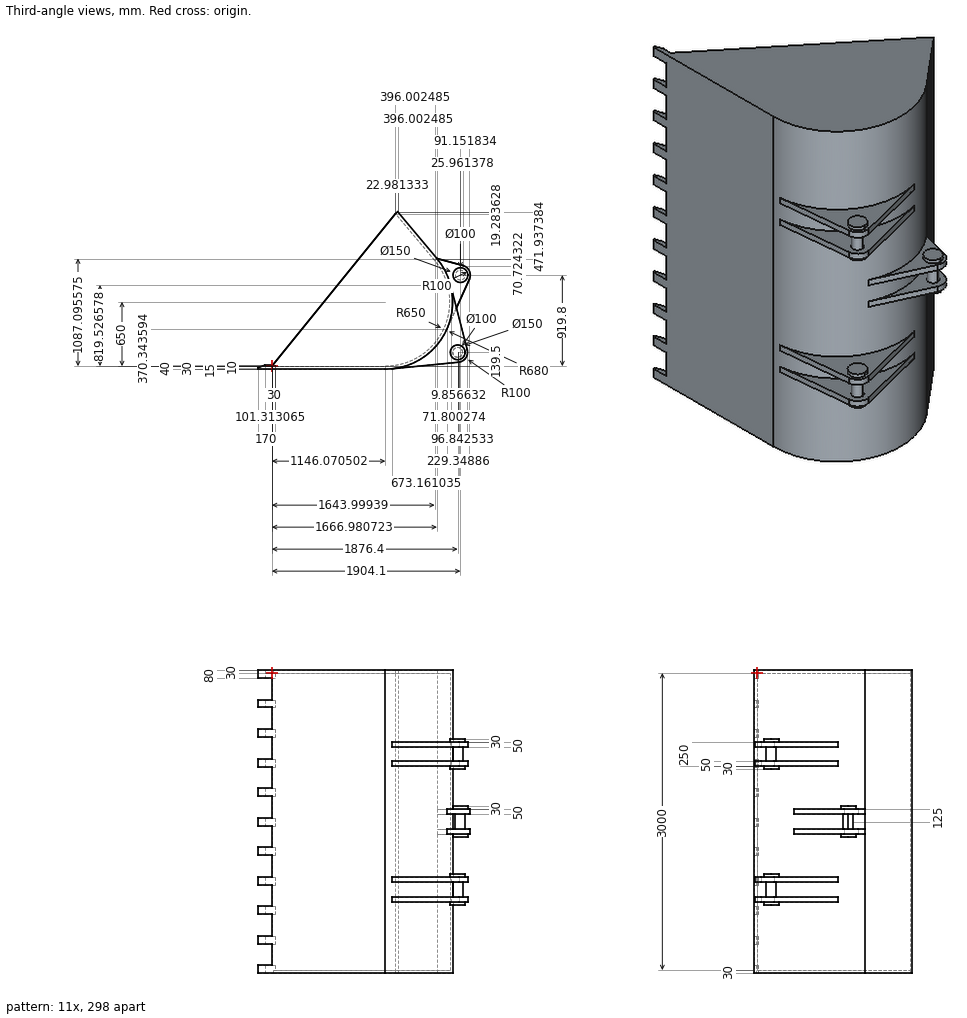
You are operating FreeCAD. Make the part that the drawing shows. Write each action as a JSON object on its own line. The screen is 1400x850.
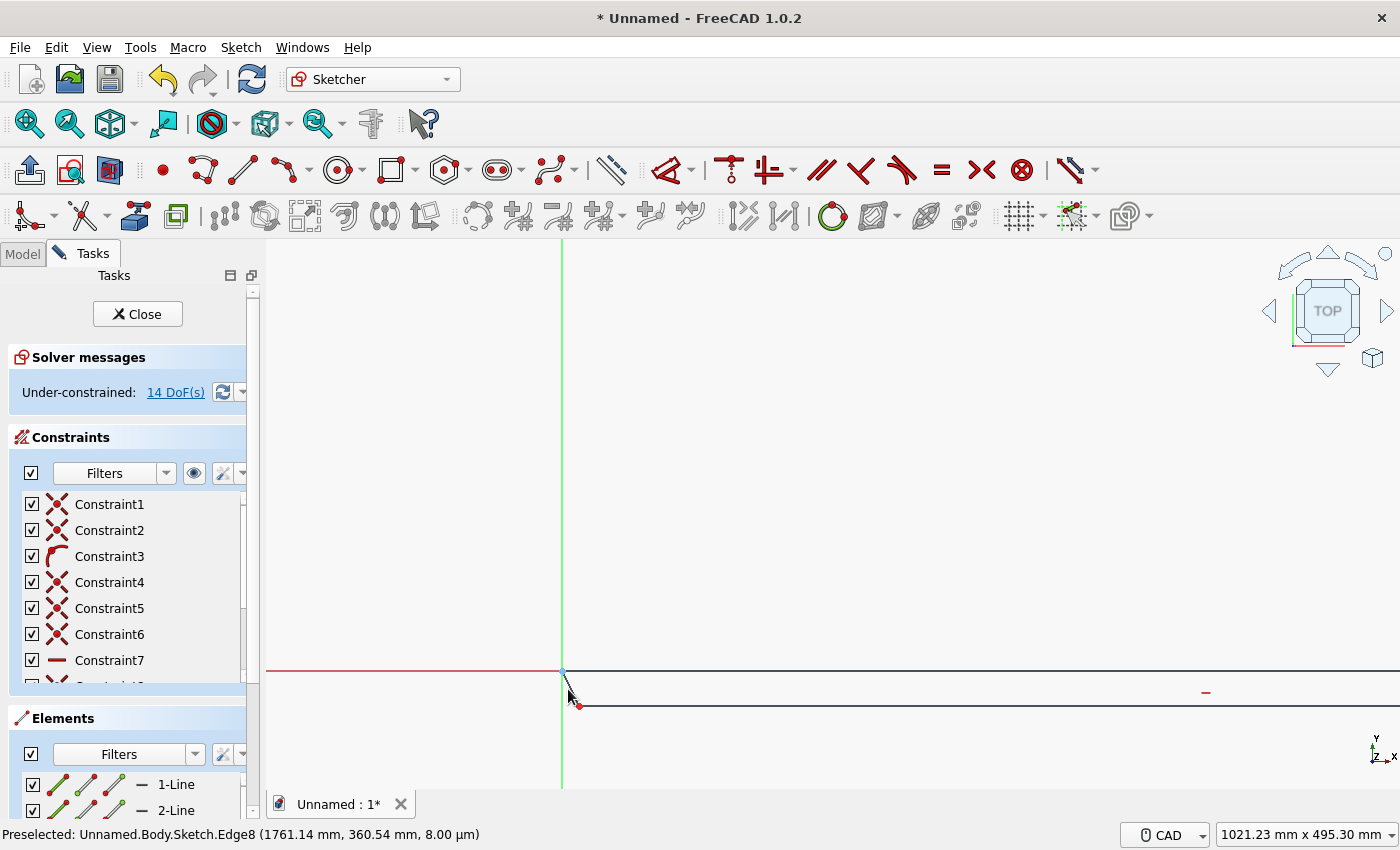
{"action": "left_click", "coordinate": [569, 685]}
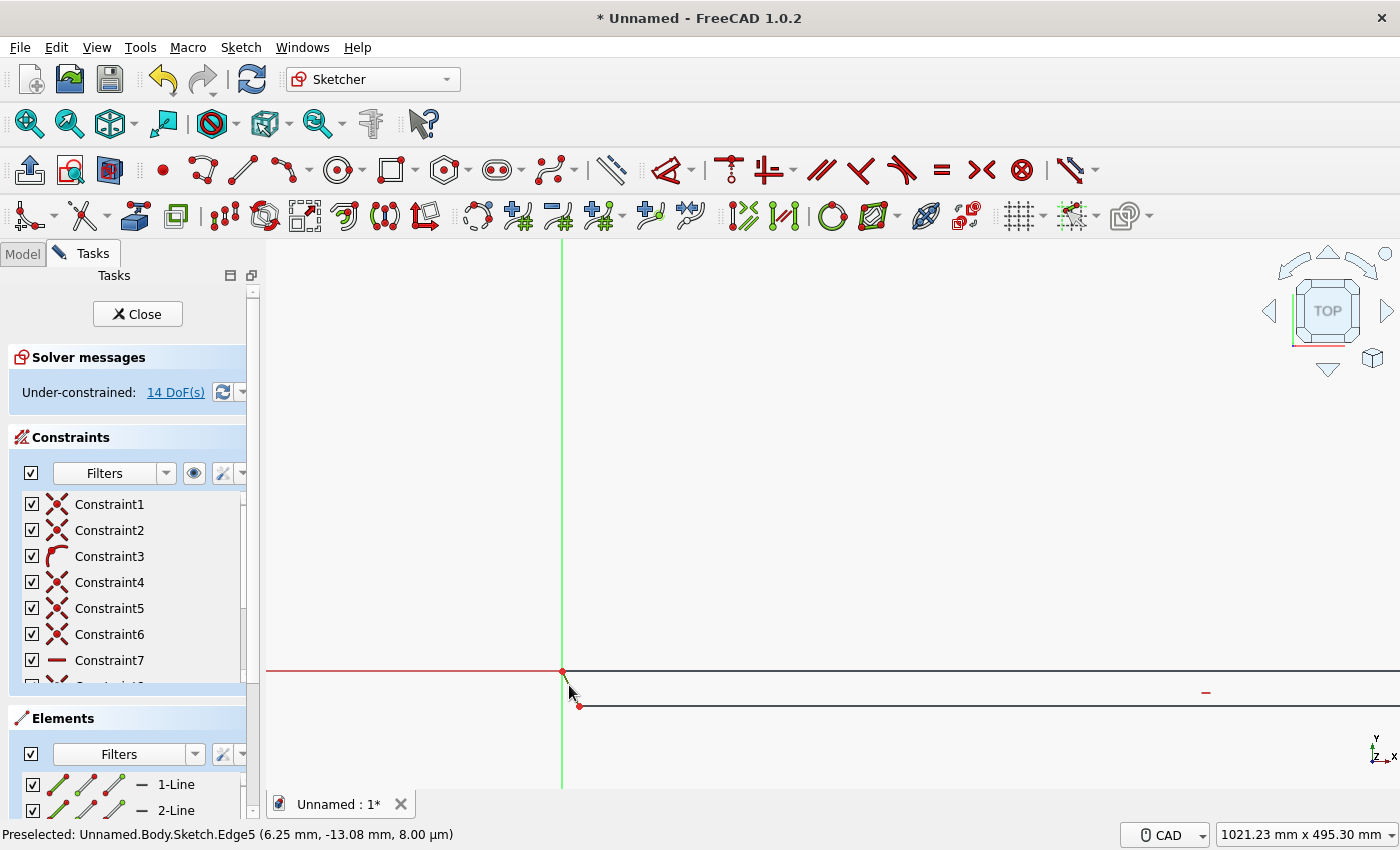
{"action": "key", "text": "v"}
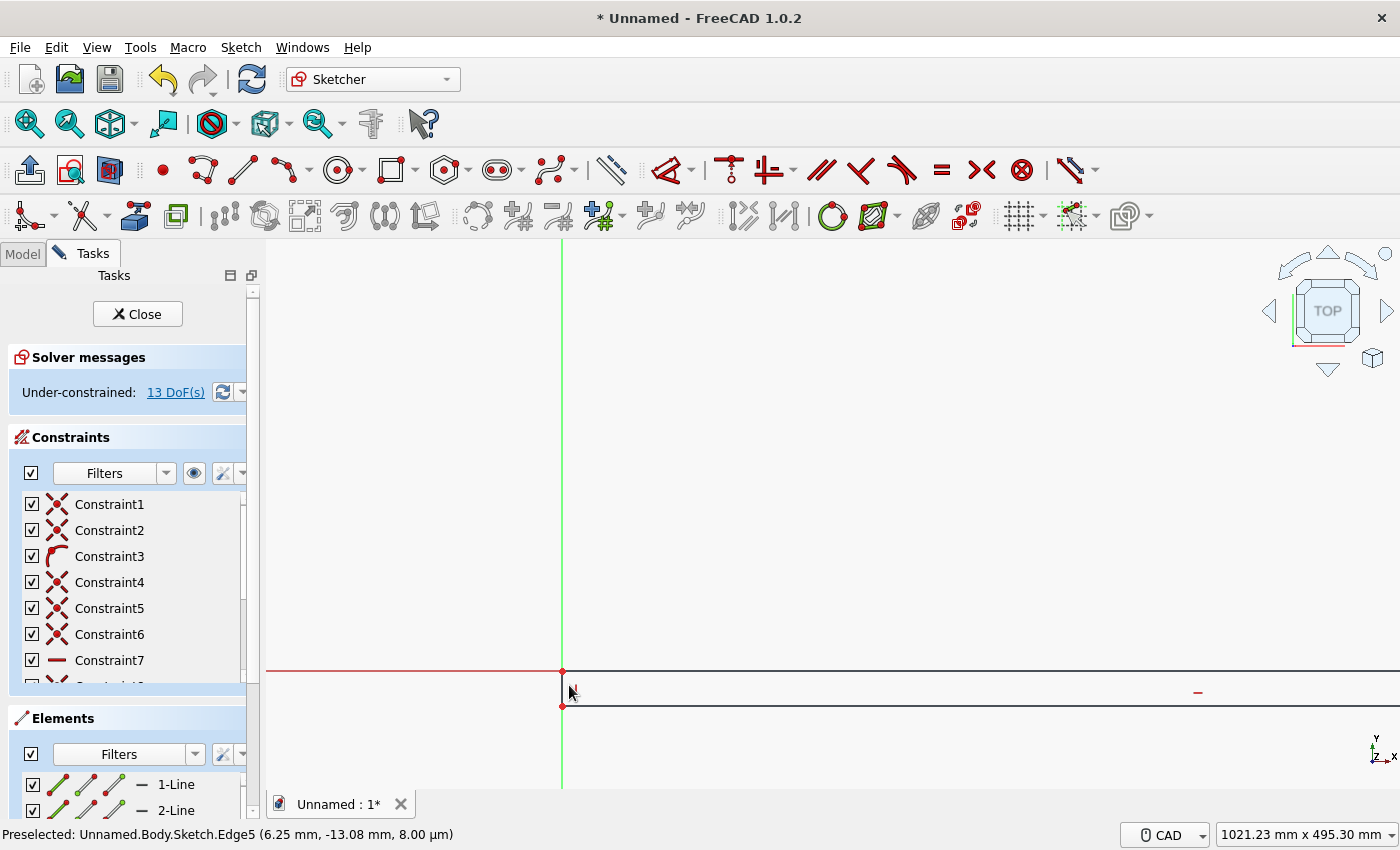
{"action": "scroll", "coordinate": [568, 689], "scroll_direction": "down", "scroll_amount": 8}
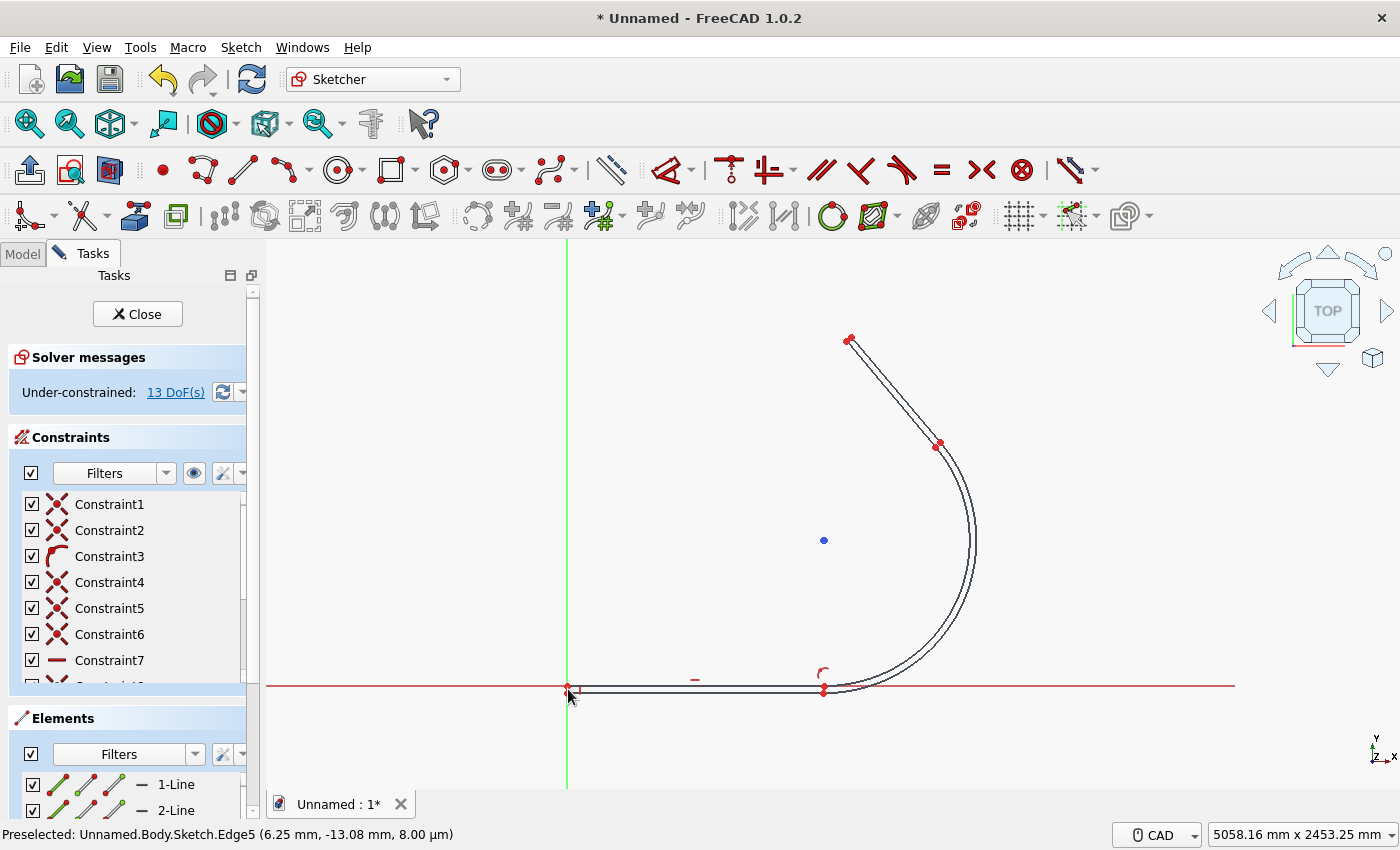
{"action": "scroll", "coordinate": [916, 654], "scroll_direction": "up", "scroll_amount": 4}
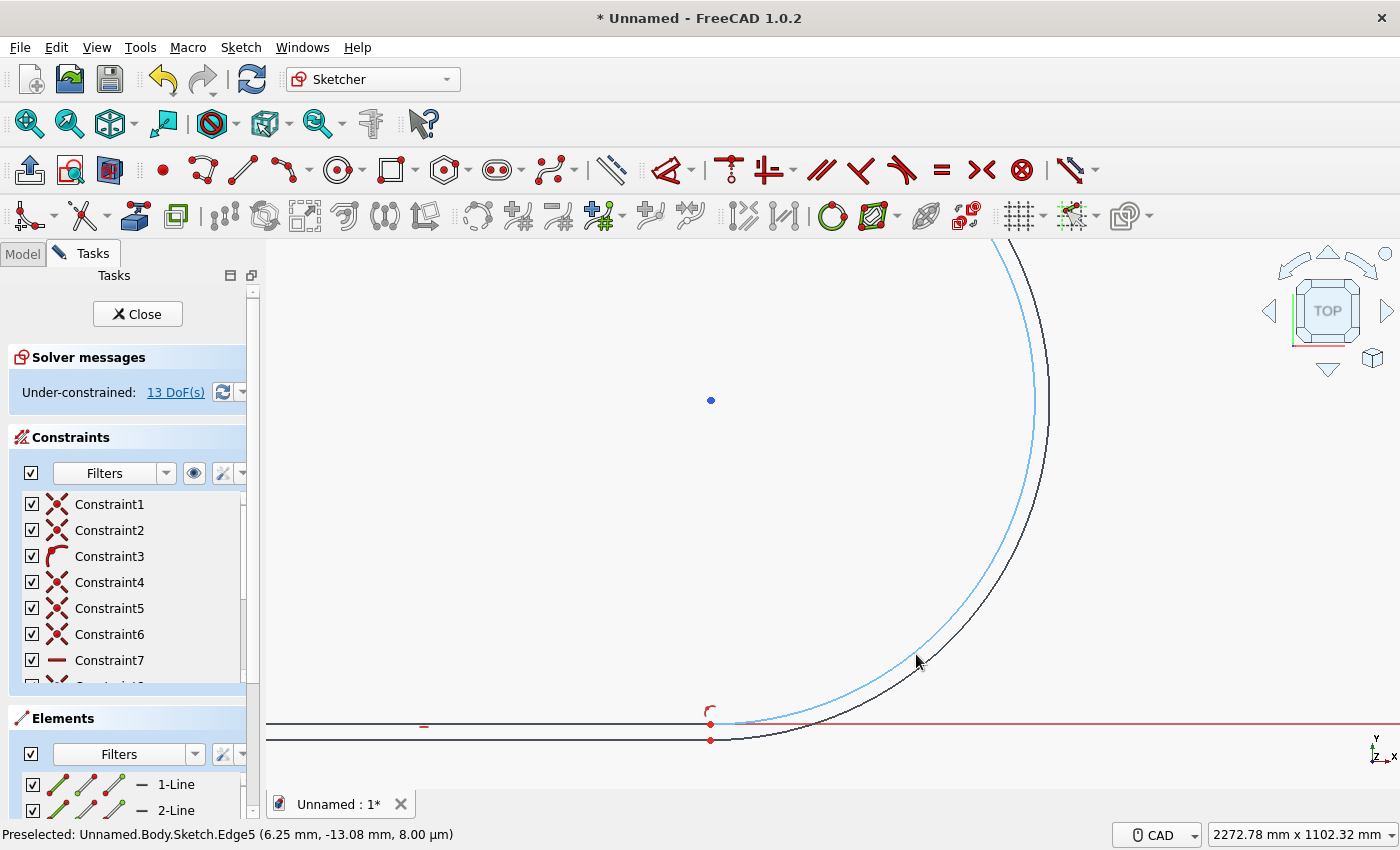
{"action": "left_click", "coordinate": [915, 653]}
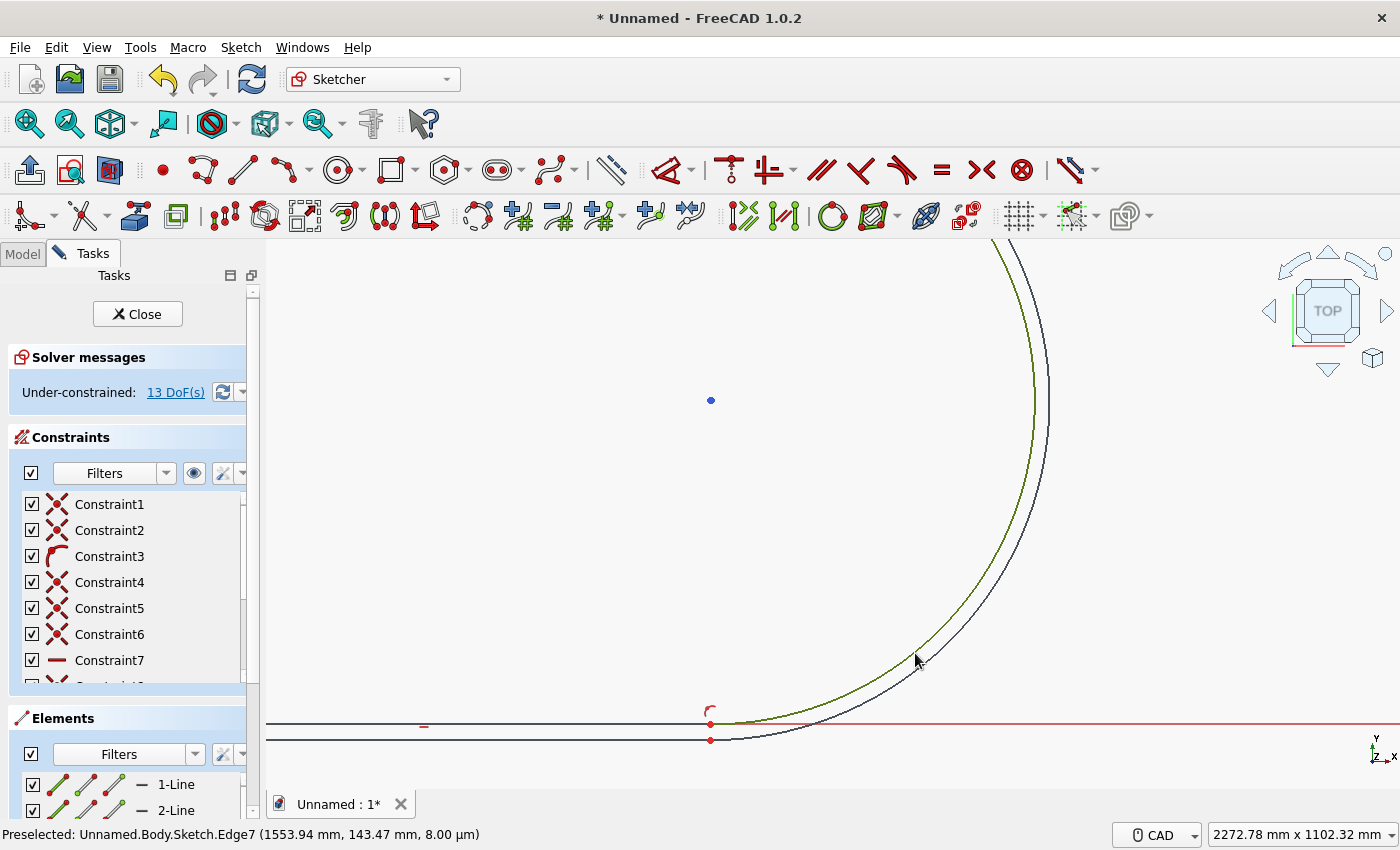
{"action": "left_click", "coordinate": [924, 665]}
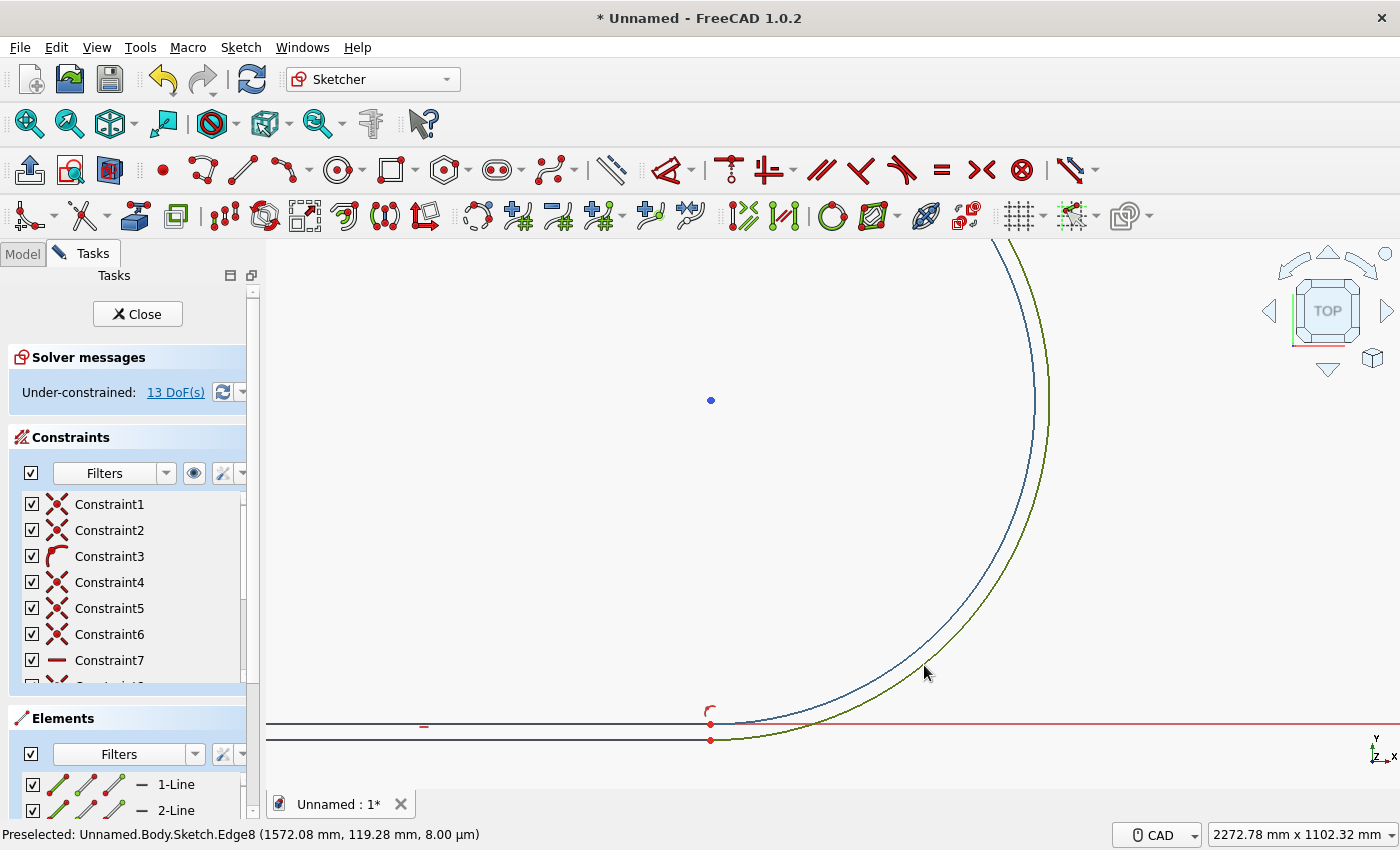
{"action": "left_click", "coordinate": [730, 170]}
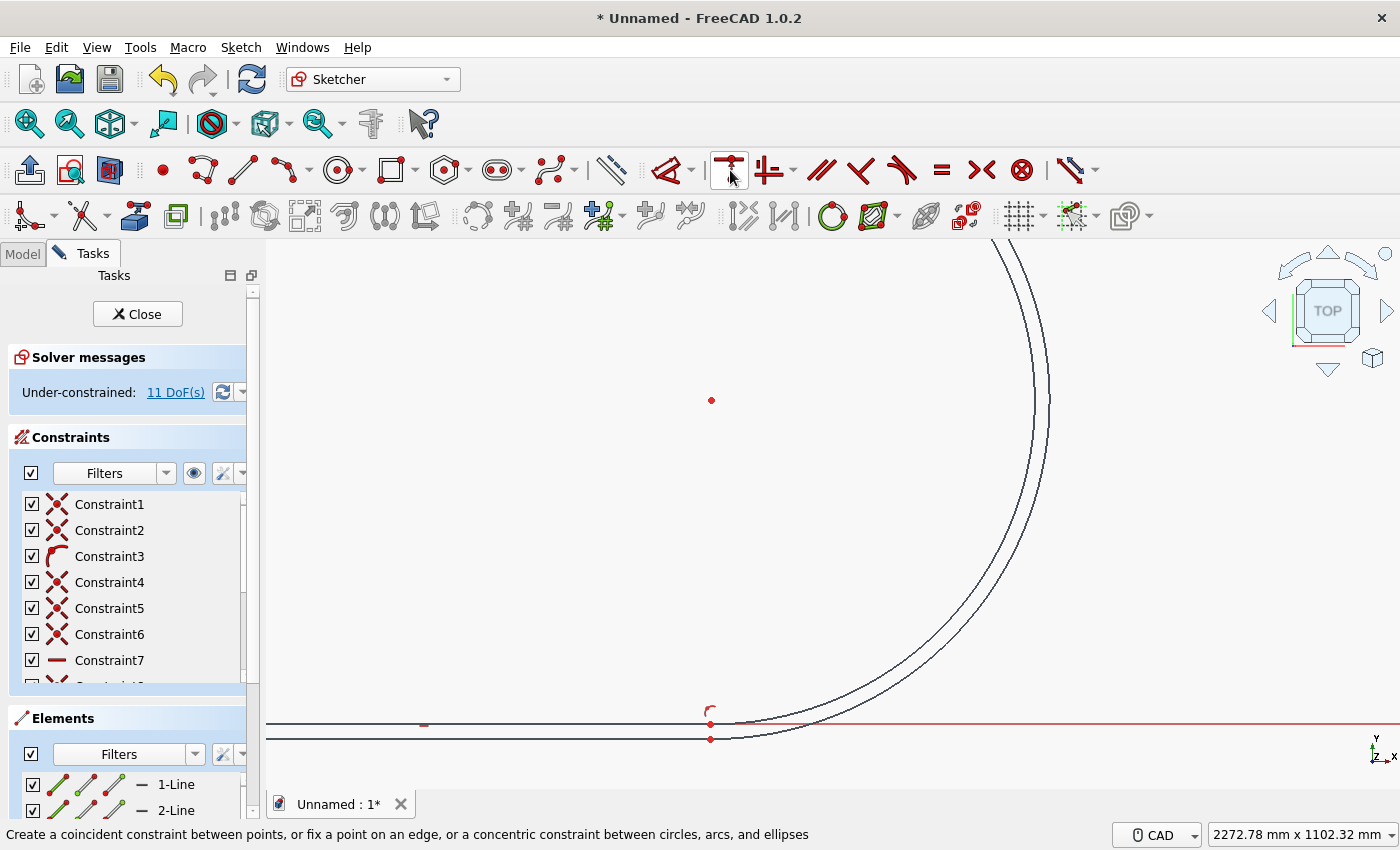
{"action": "left_click", "coordinate": [666, 170]}